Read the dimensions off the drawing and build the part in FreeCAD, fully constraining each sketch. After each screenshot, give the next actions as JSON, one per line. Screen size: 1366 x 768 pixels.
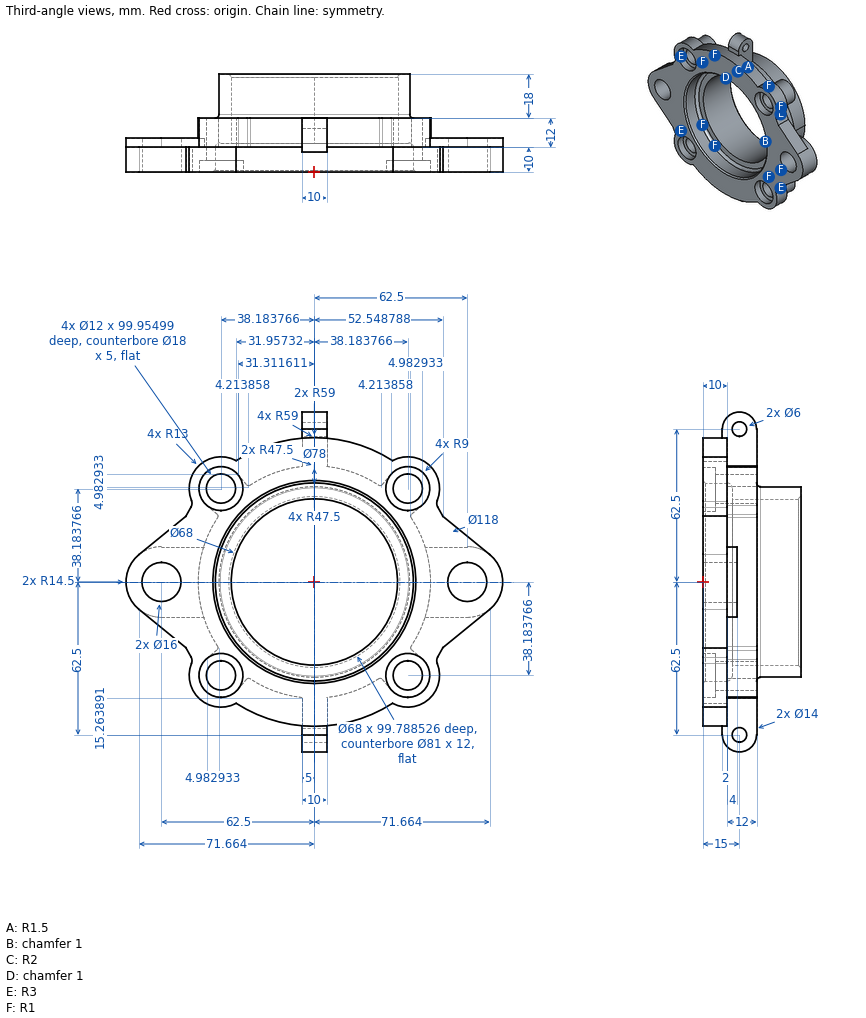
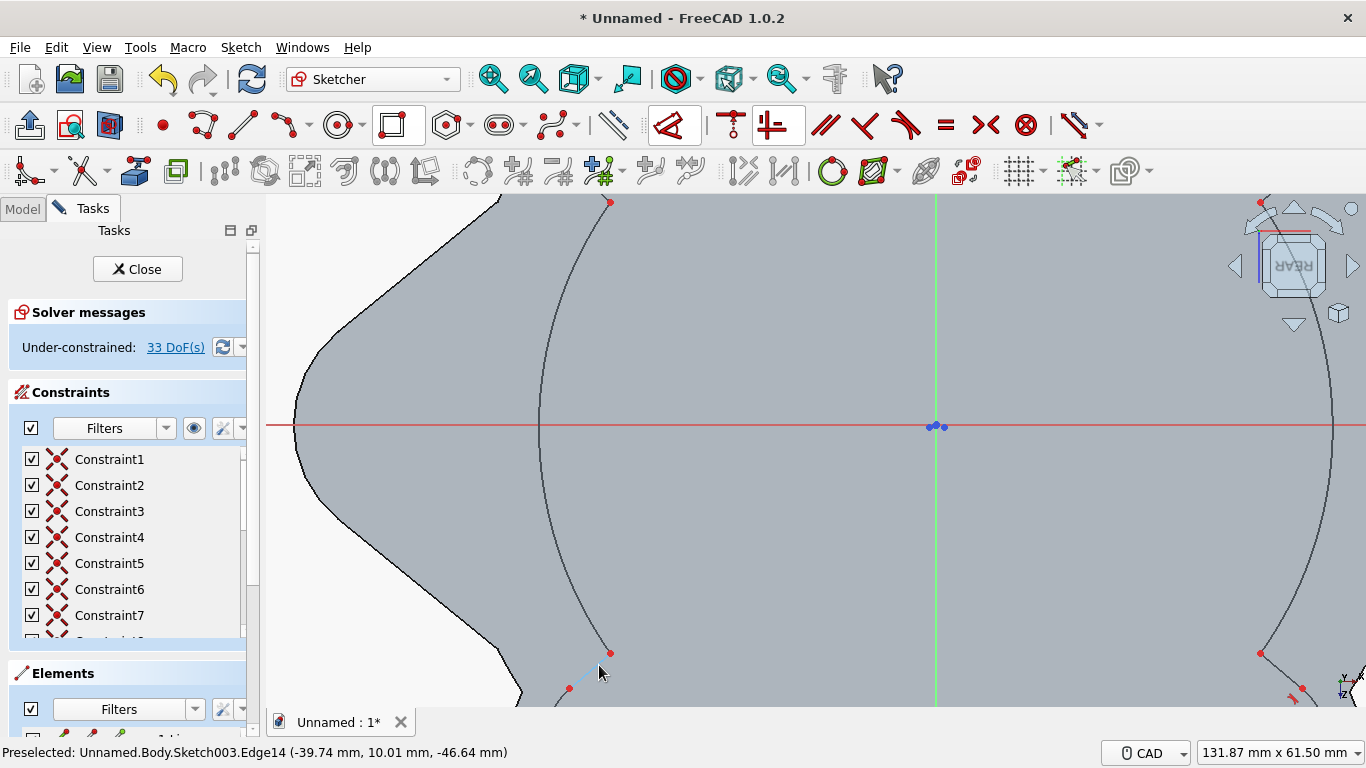
{"action": "left_click", "coordinate": [598, 664]}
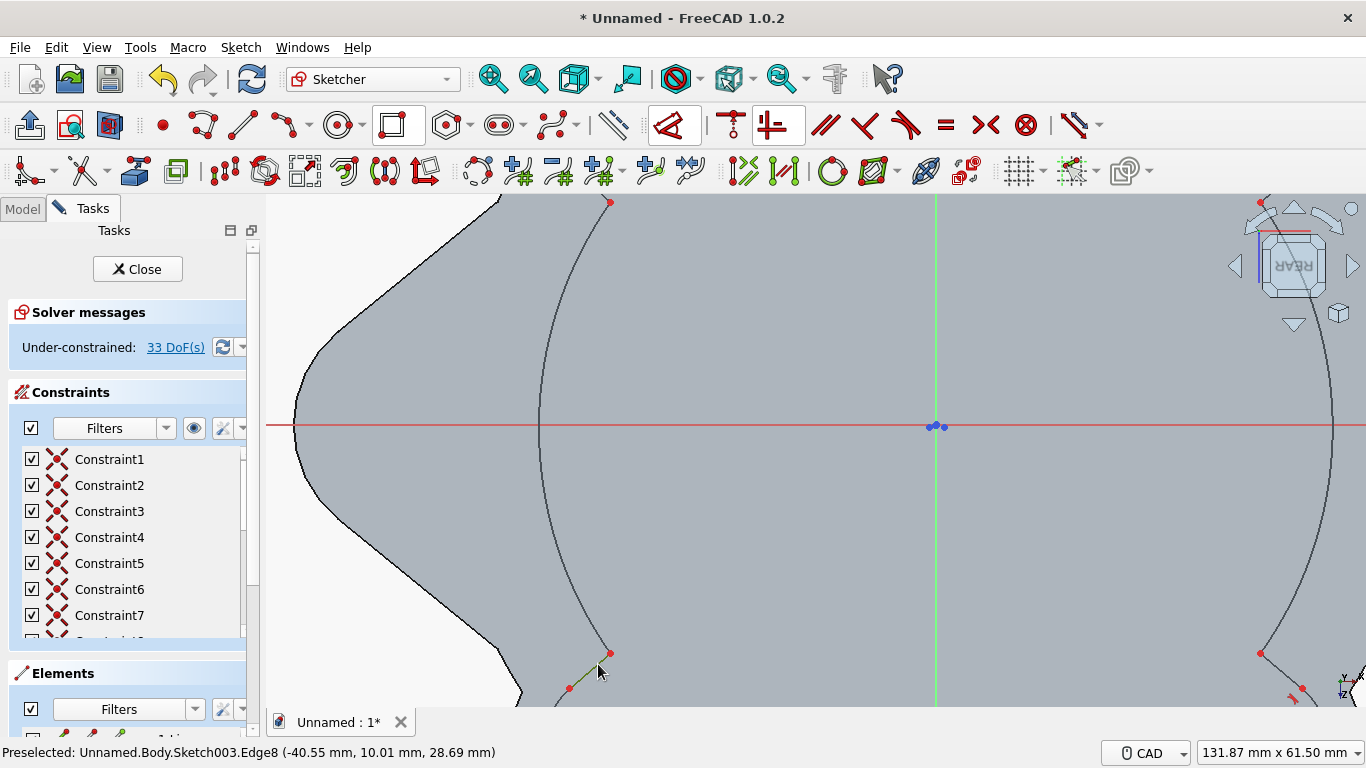
{"action": "scroll", "coordinate": [594, 471], "scroll_direction": "down", "scroll_amount": 4}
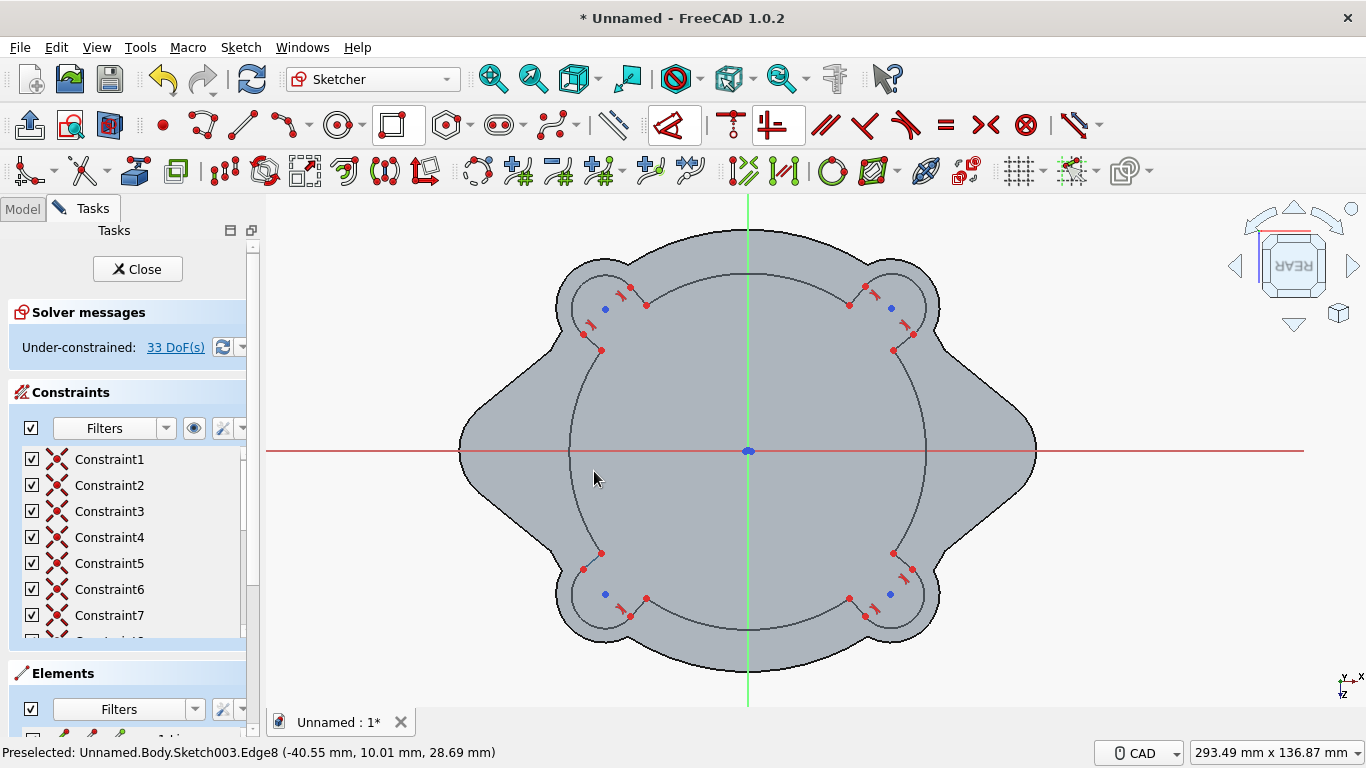
{"action": "left_click", "coordinate": [572, 599]}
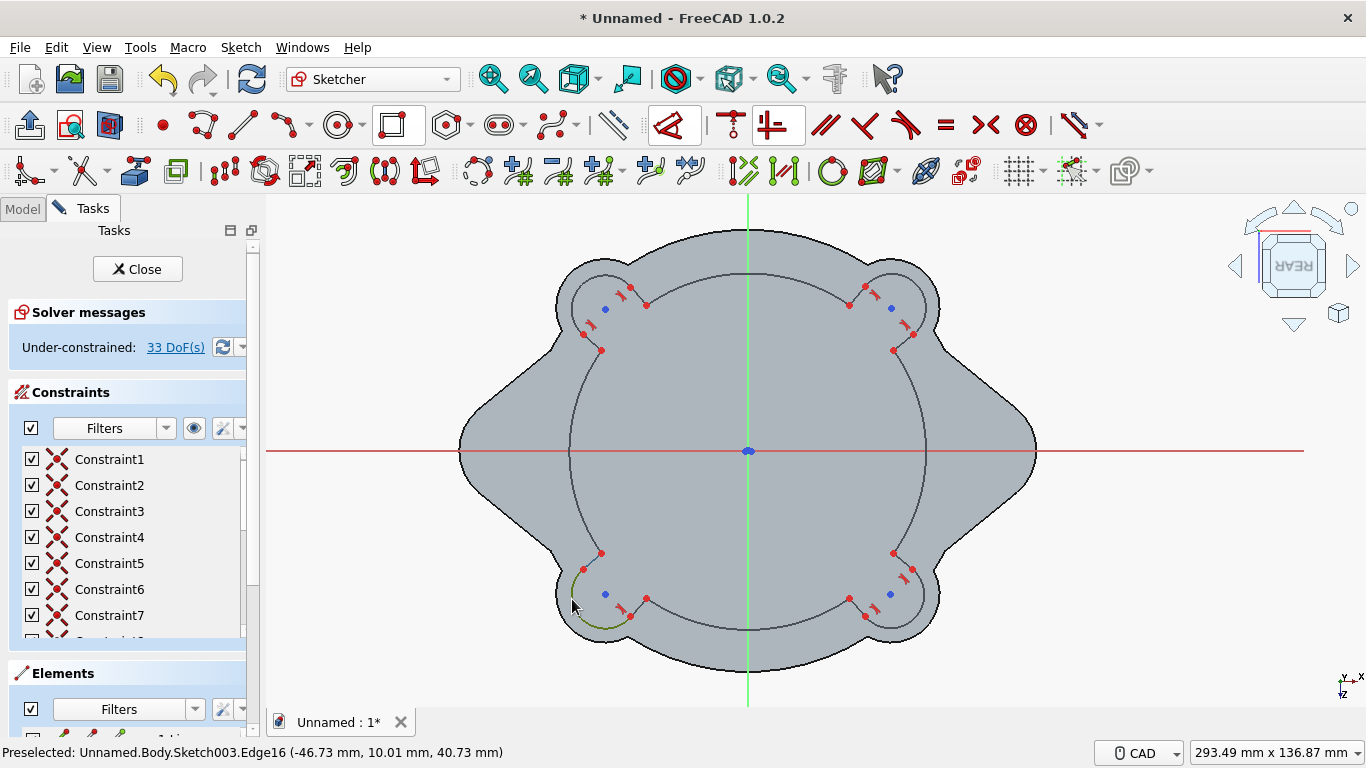
{"action": "left_click", "coordinate": [906, 126]}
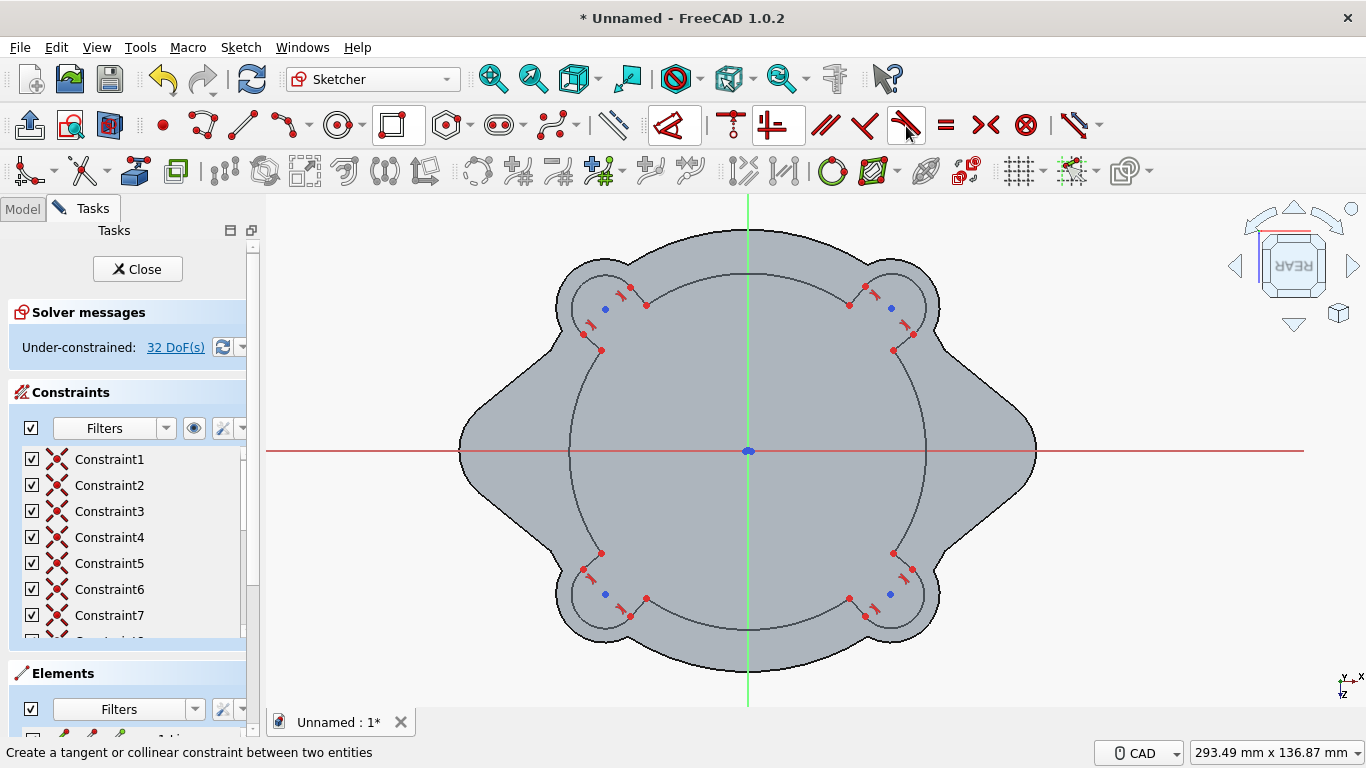
{"action": "left_click", "coordinate": [706, 625]}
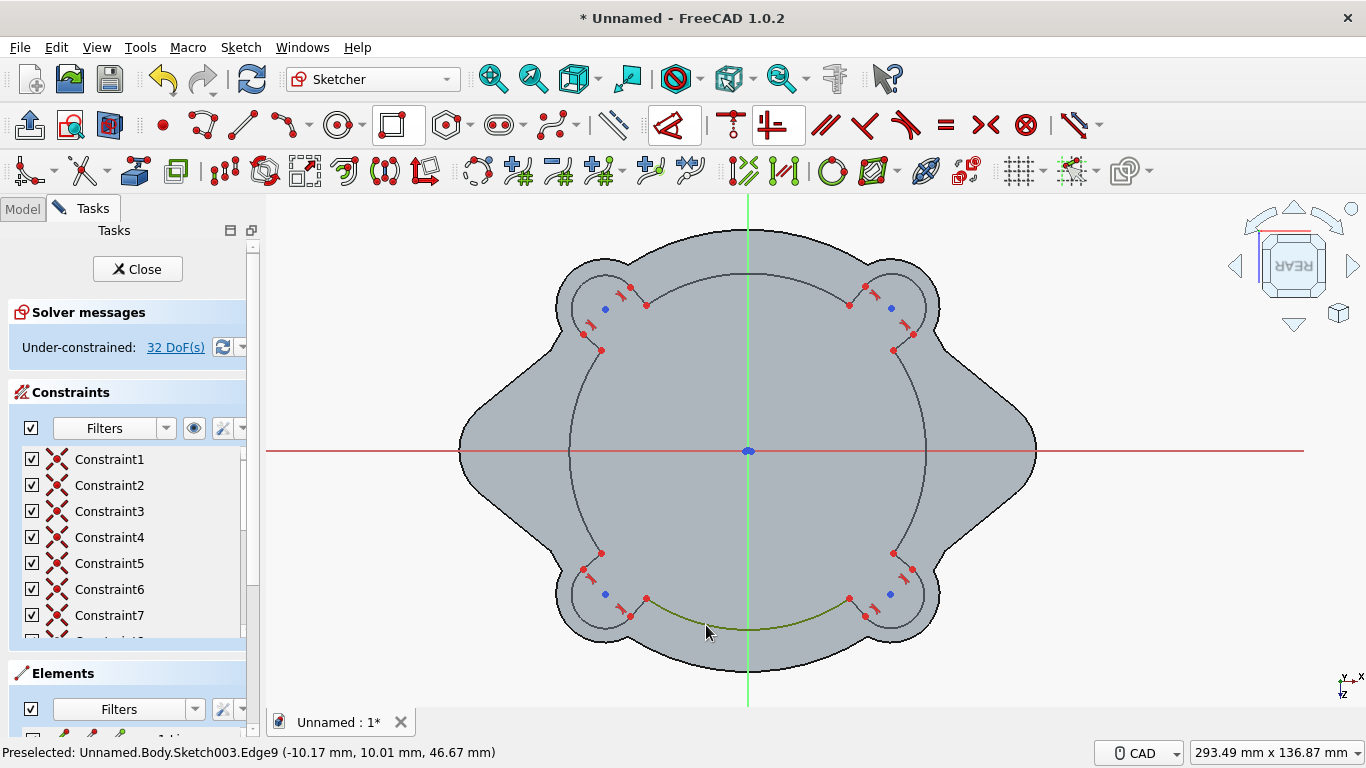
{"action": "left_click", "coordinate": [921, 495]}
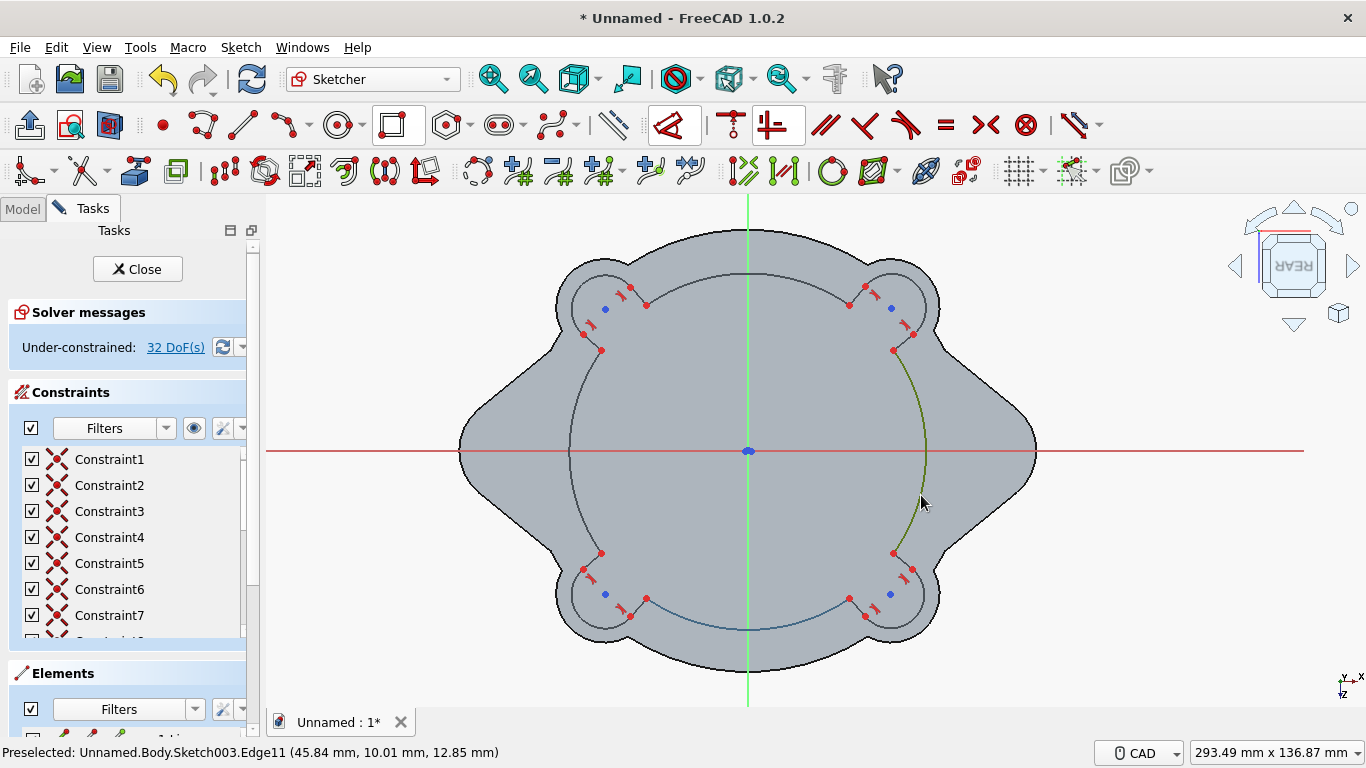
{"action": "left_click", "coordinate": [732, 126]}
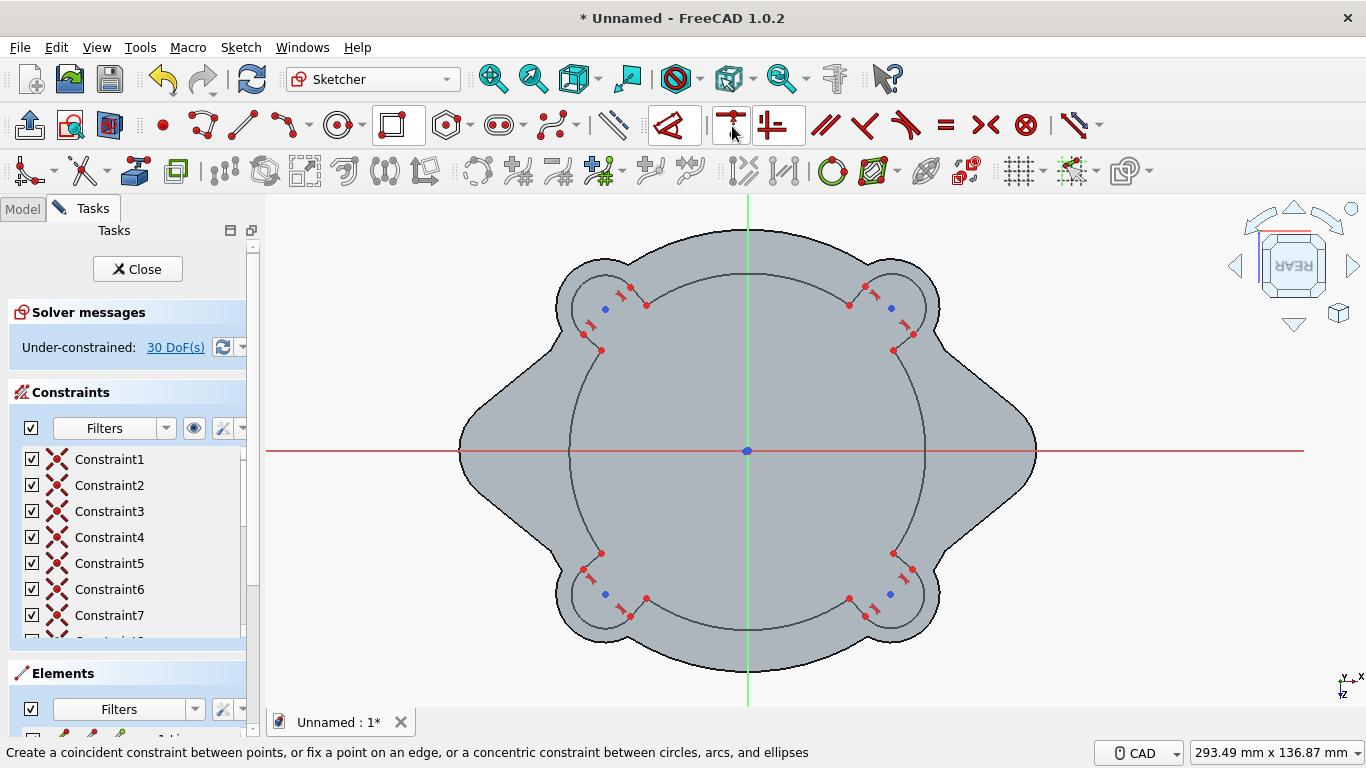
{"action": "left_click", "coordinate": [705, 625]}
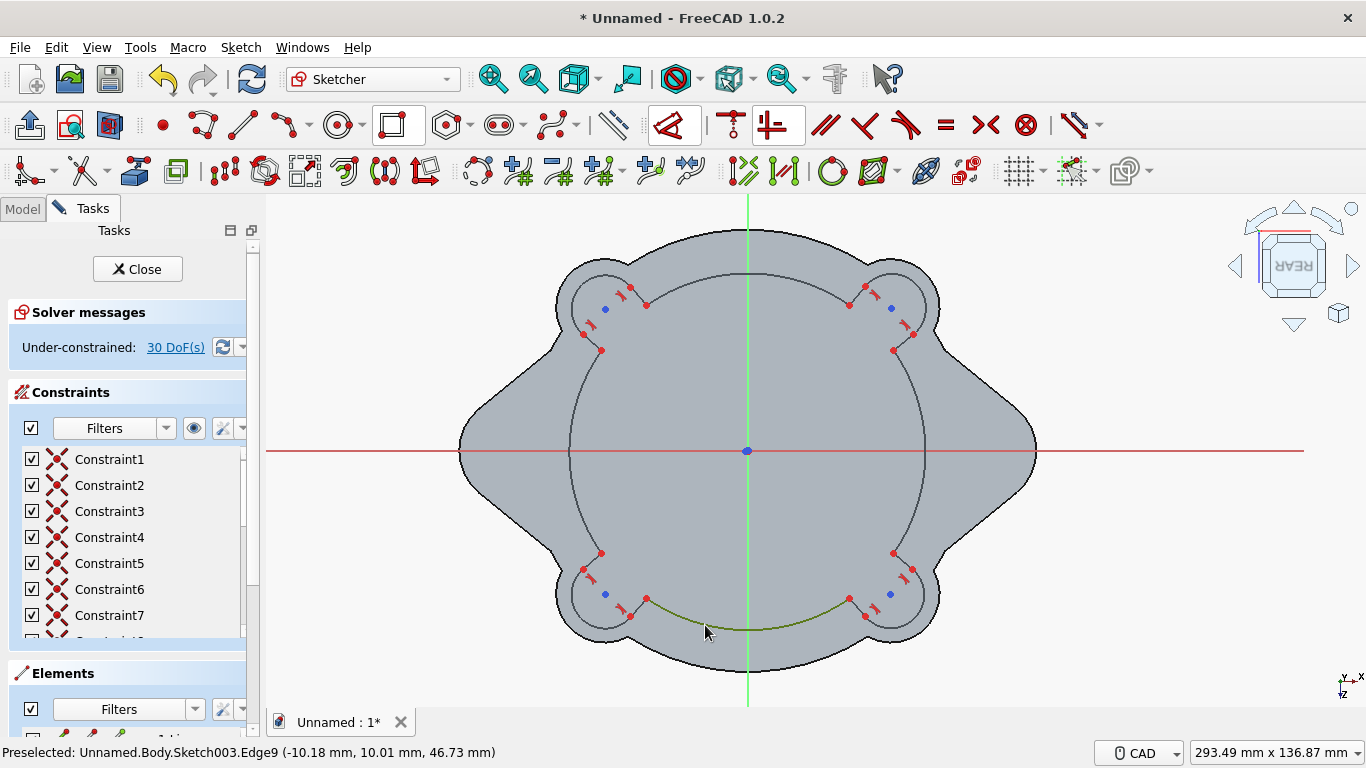
{"action": "left_click", "coordinate": [791, 279]}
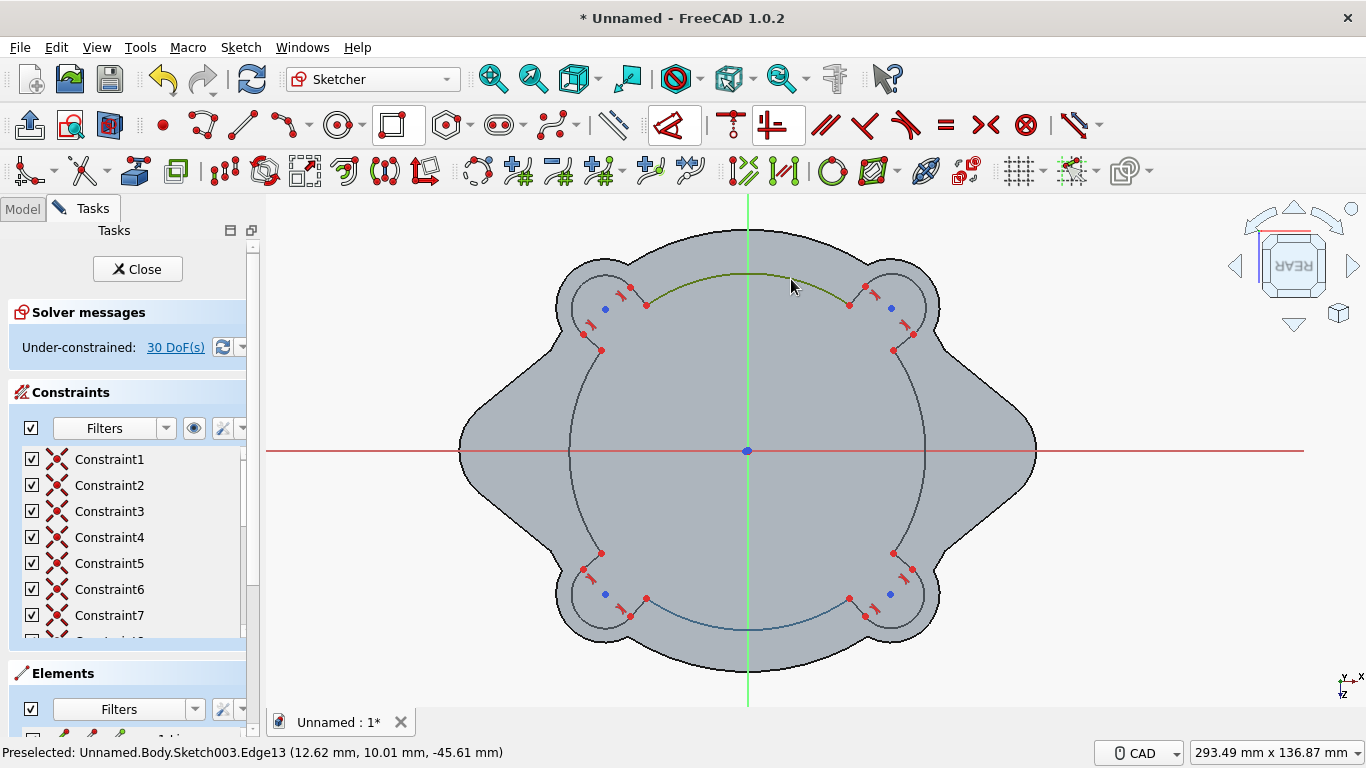
{"action": "left_click", "coordinate": [732, 126]}